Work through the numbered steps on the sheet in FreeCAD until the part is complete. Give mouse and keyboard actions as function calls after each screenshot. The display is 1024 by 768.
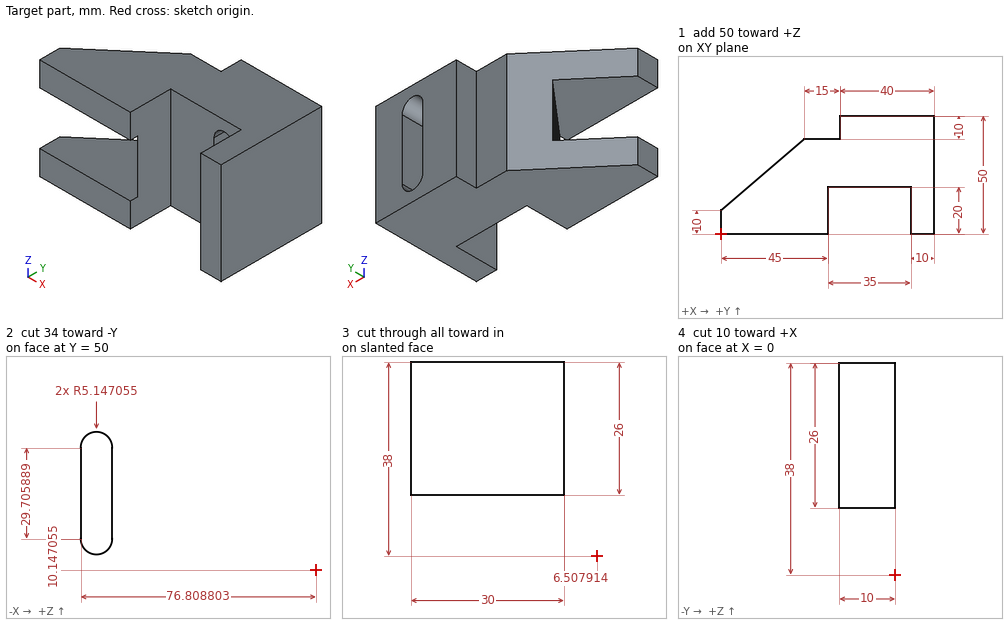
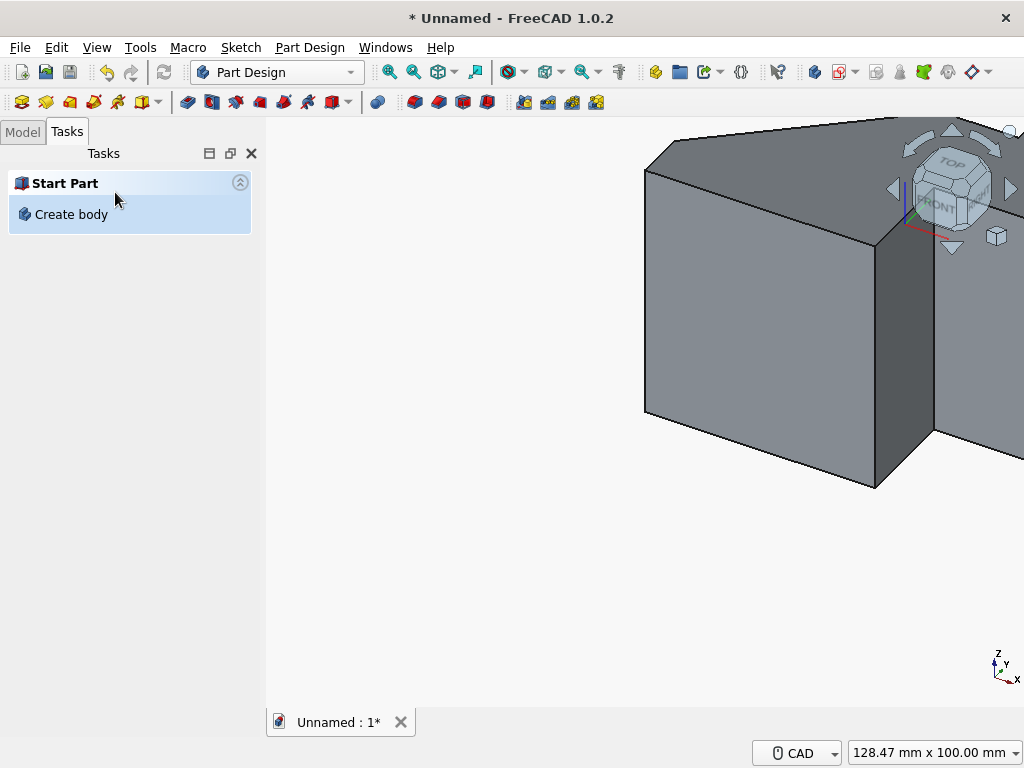
click(390, 72)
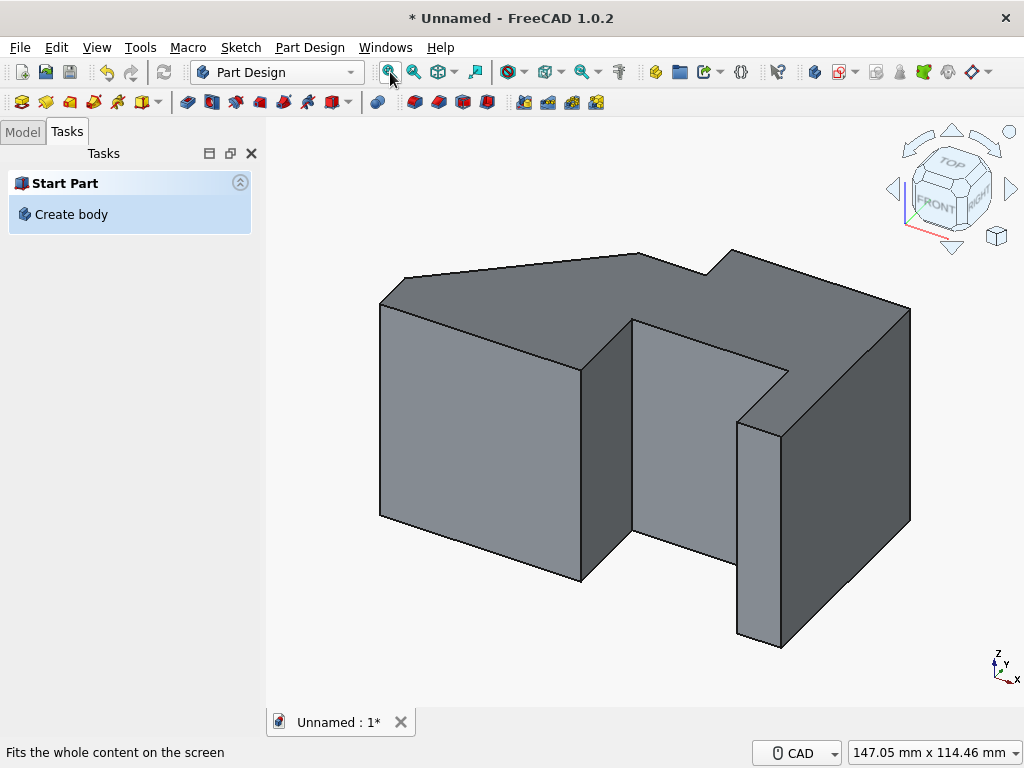
key(4)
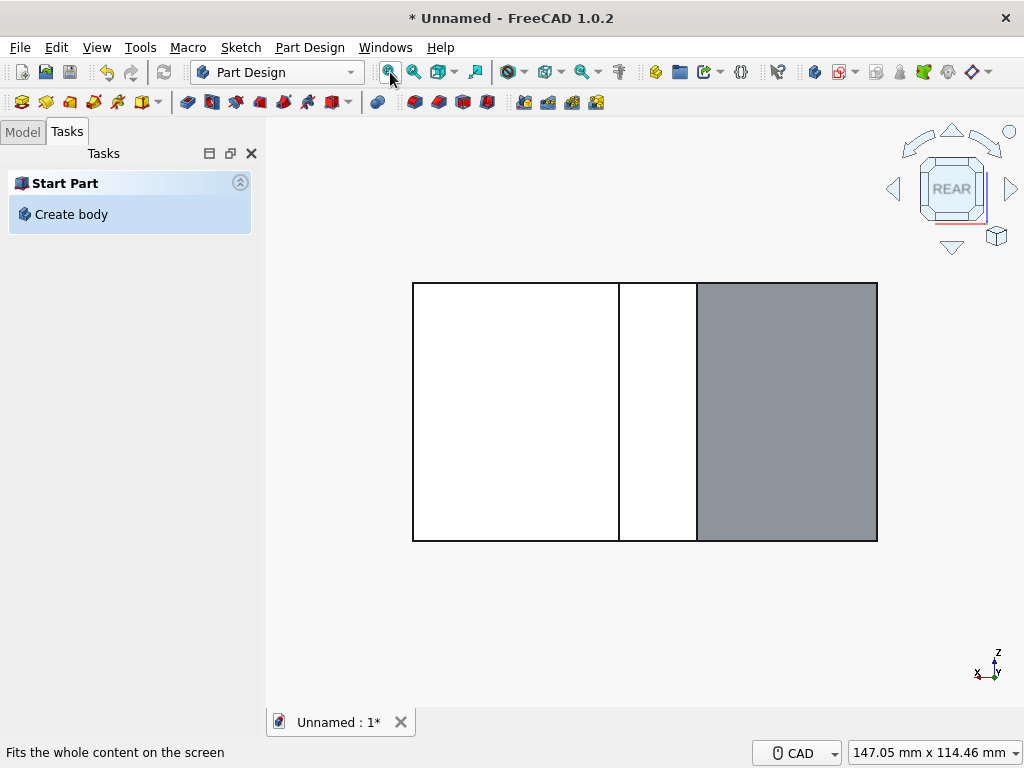
click(516, 411)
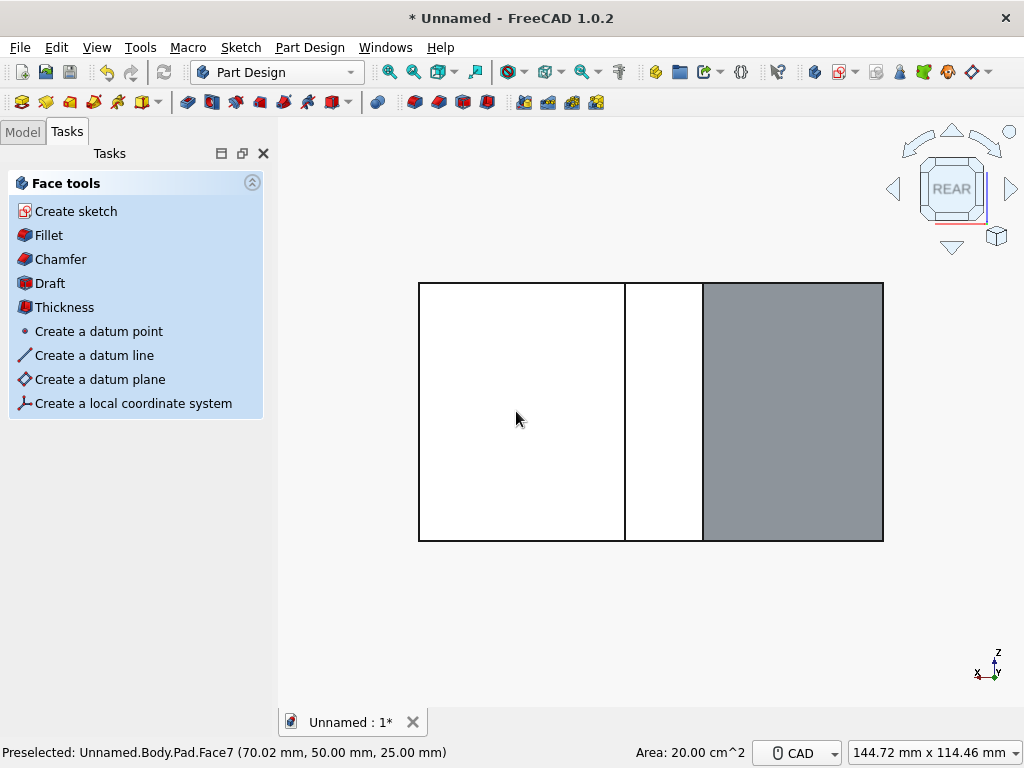
click(840, 72)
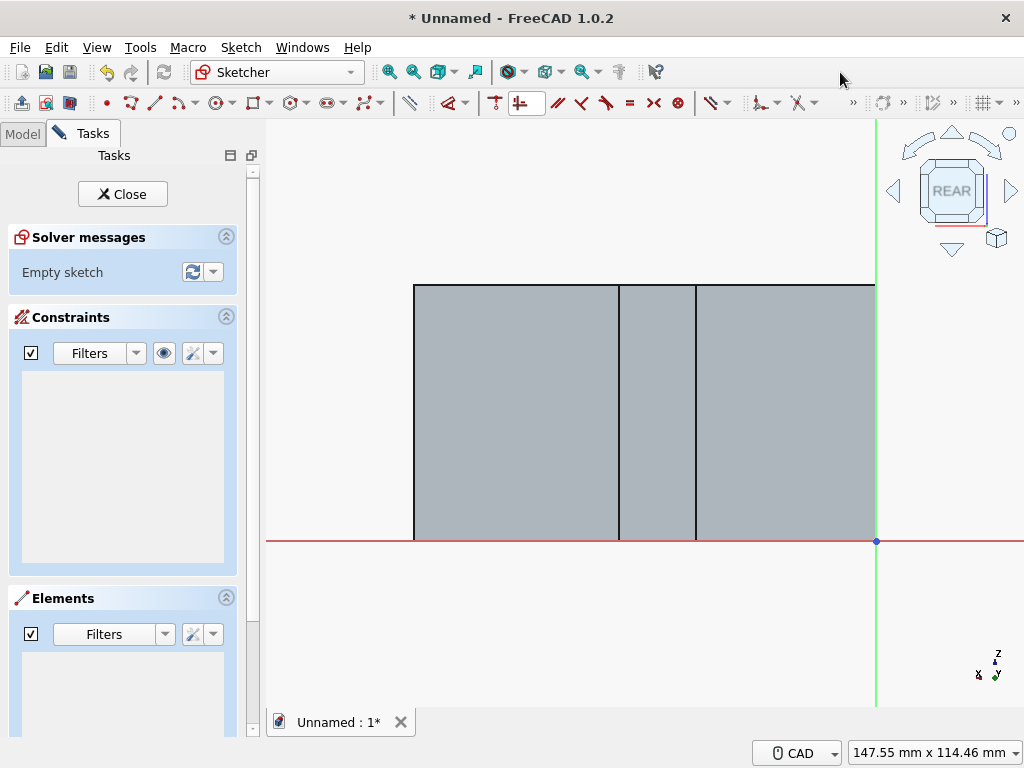
scroll(294, 355, down, 1)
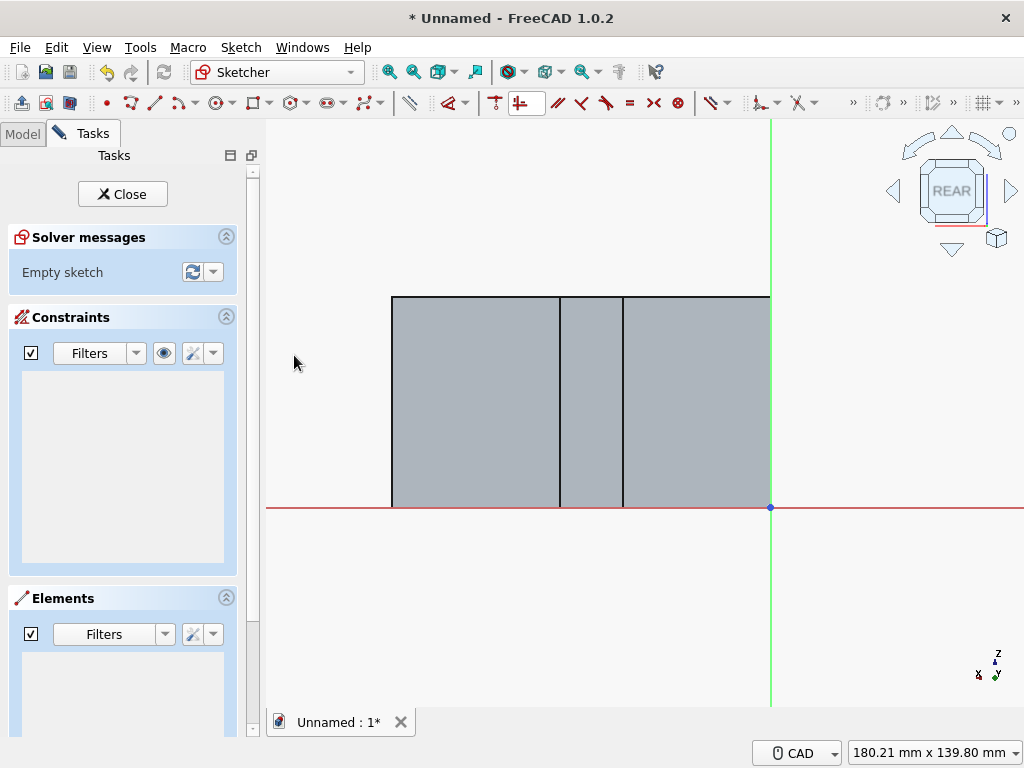
click(328, 104)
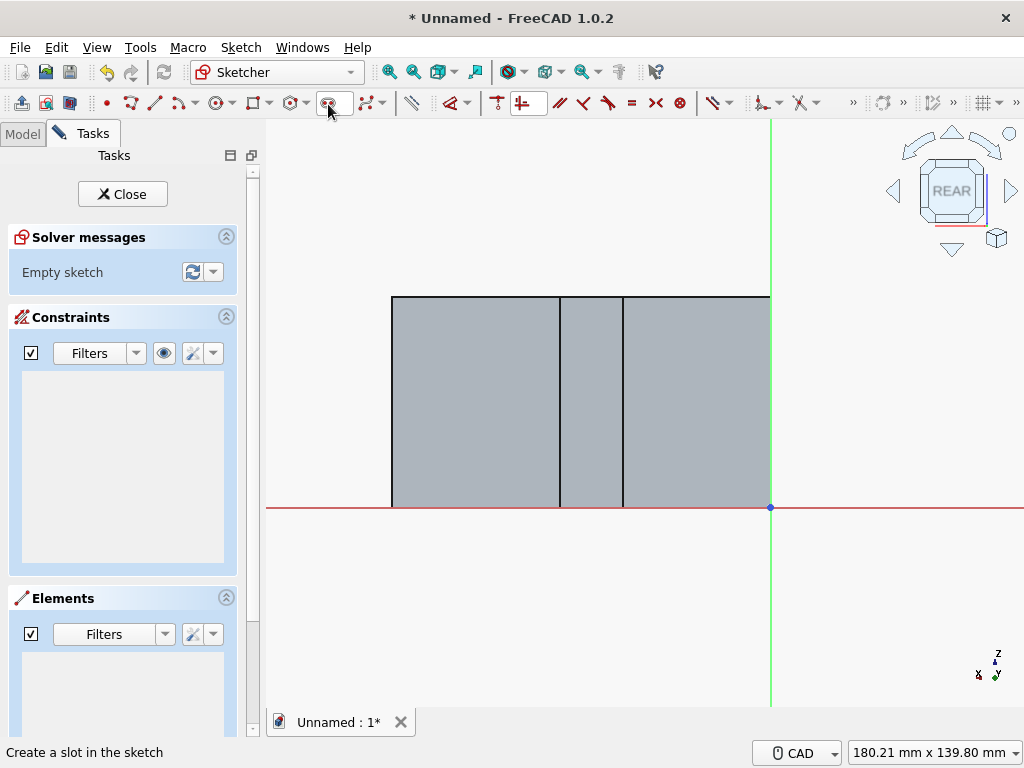
click(469, 465)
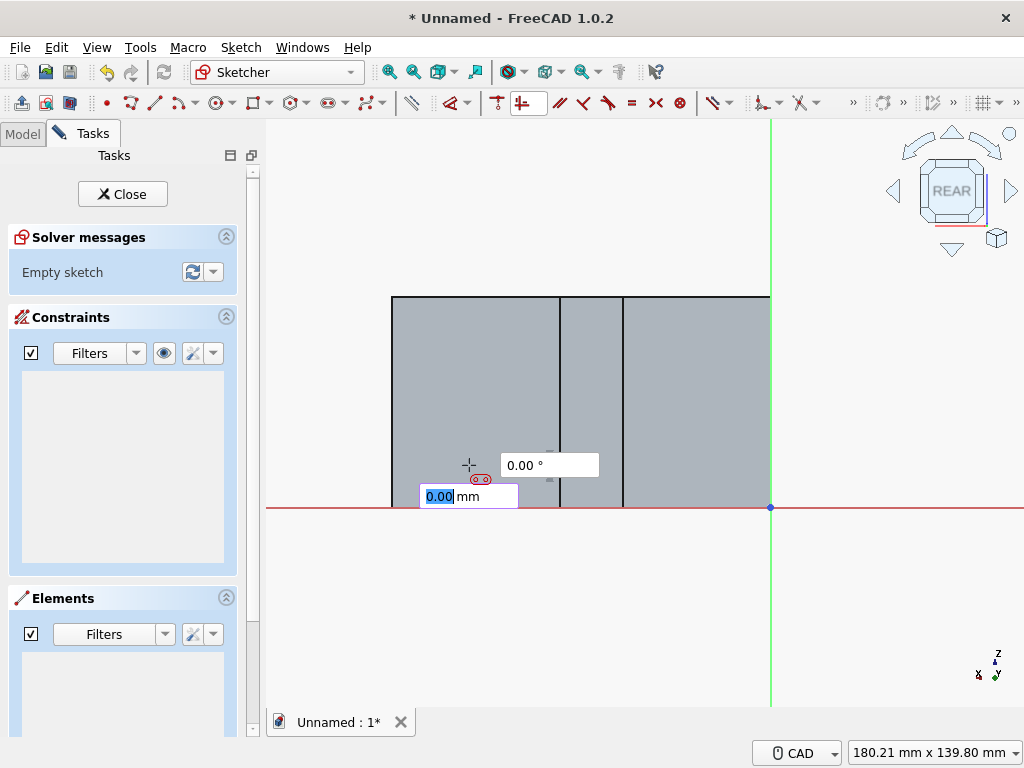
click(469, 340)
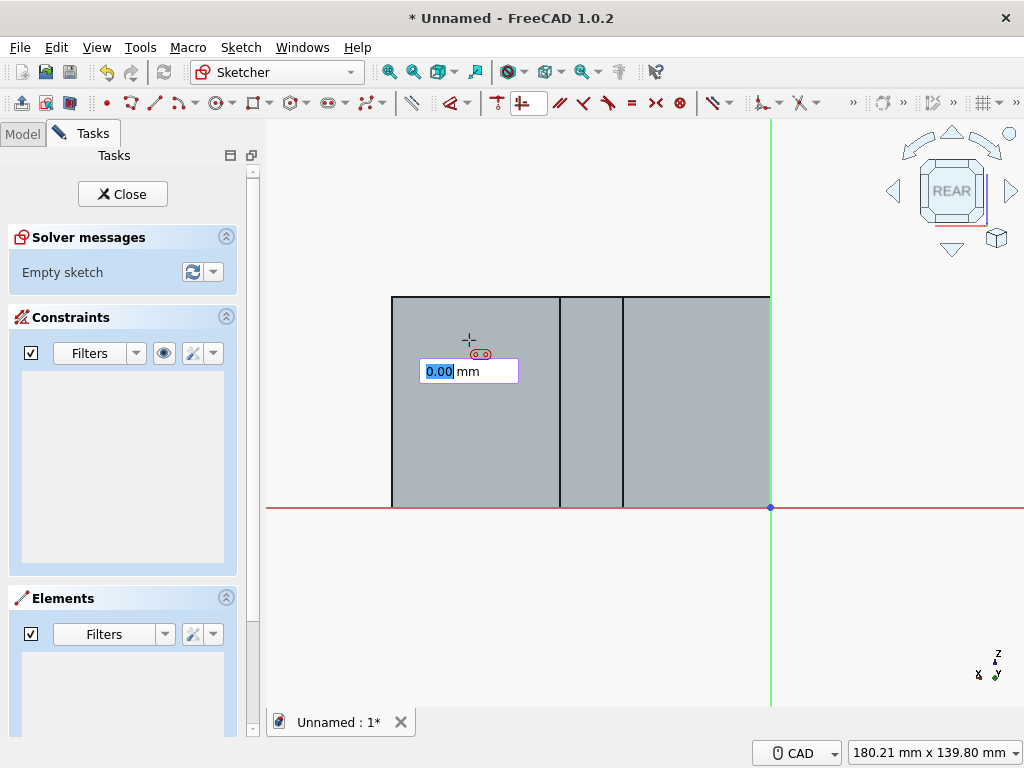
click(448, 403)
key(Escape)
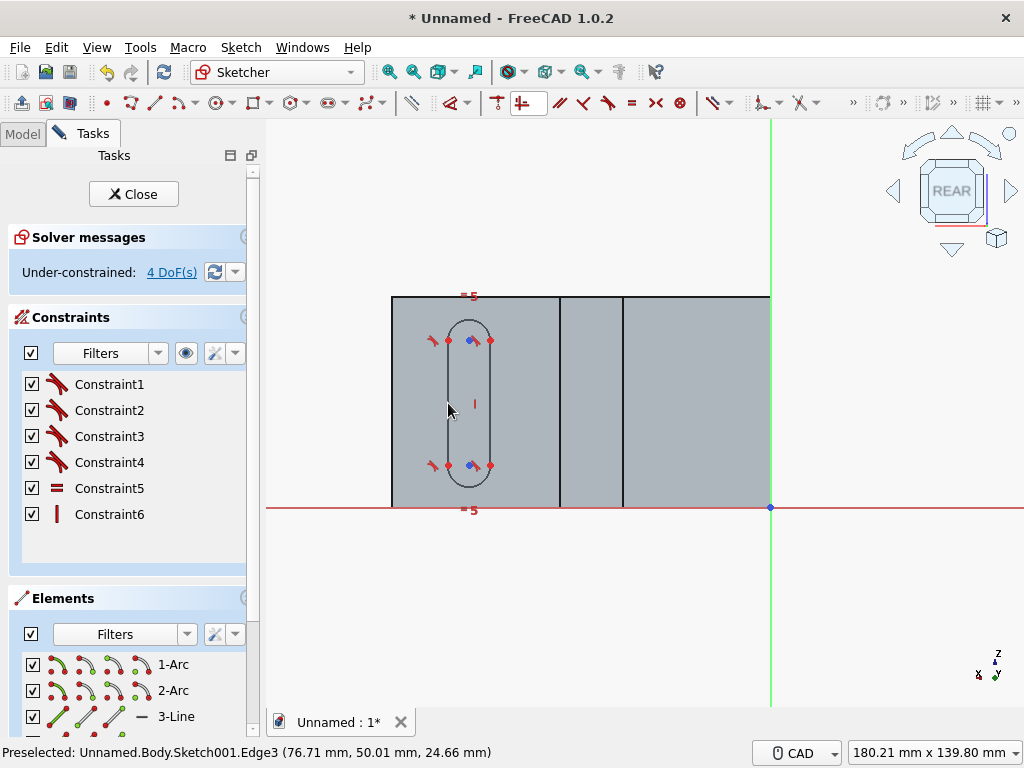
key(d)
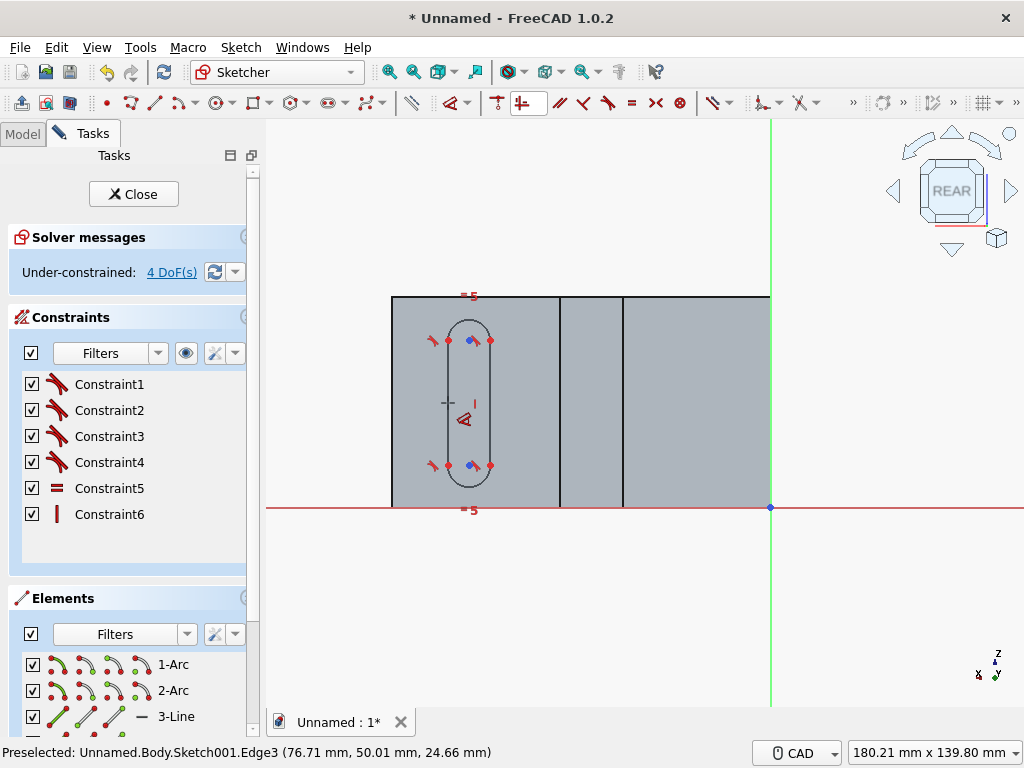
scroll(457, 483, up, 4)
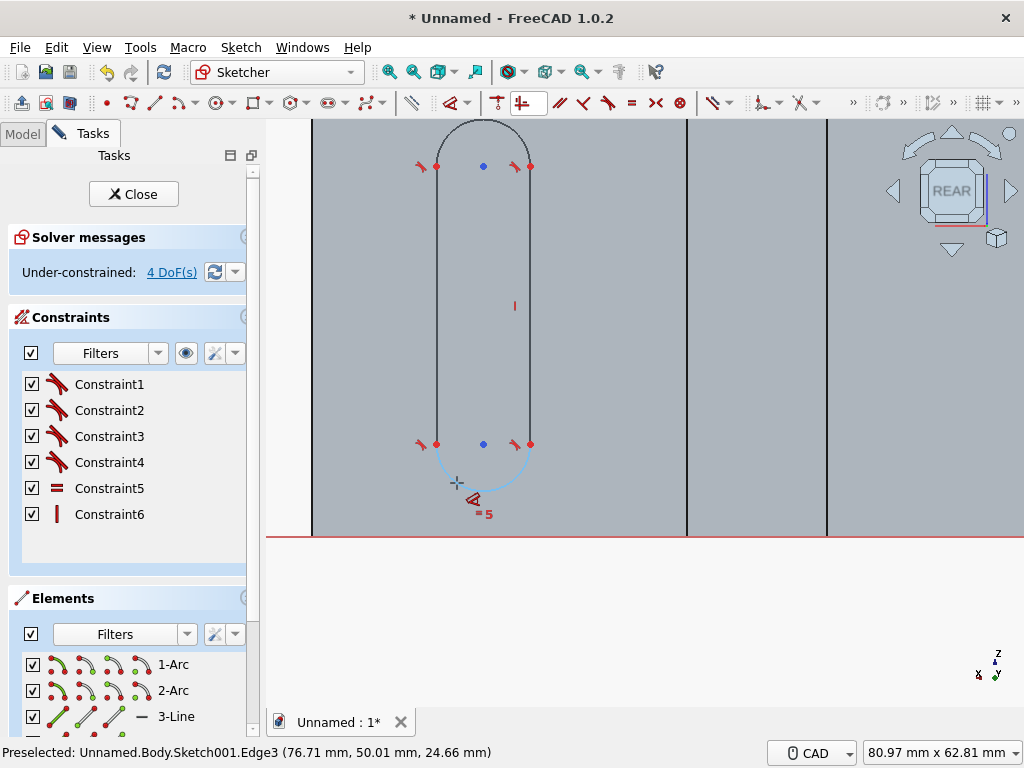
click(456, 482)
click(437, 508)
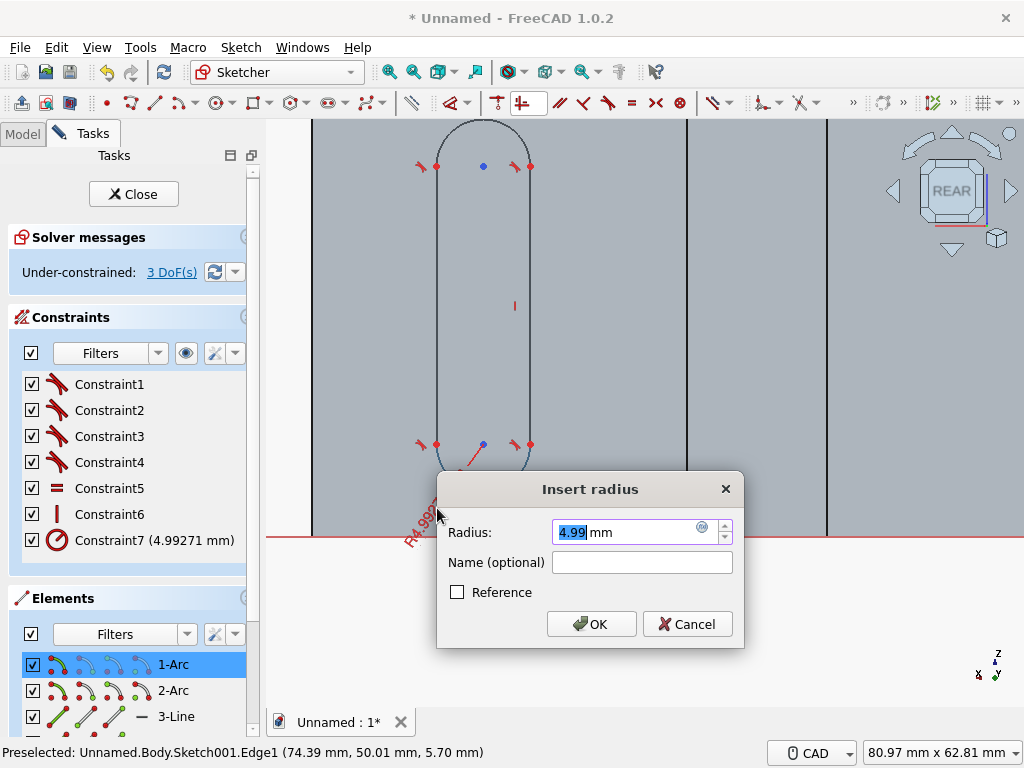
text(5.147055)
key(Return)